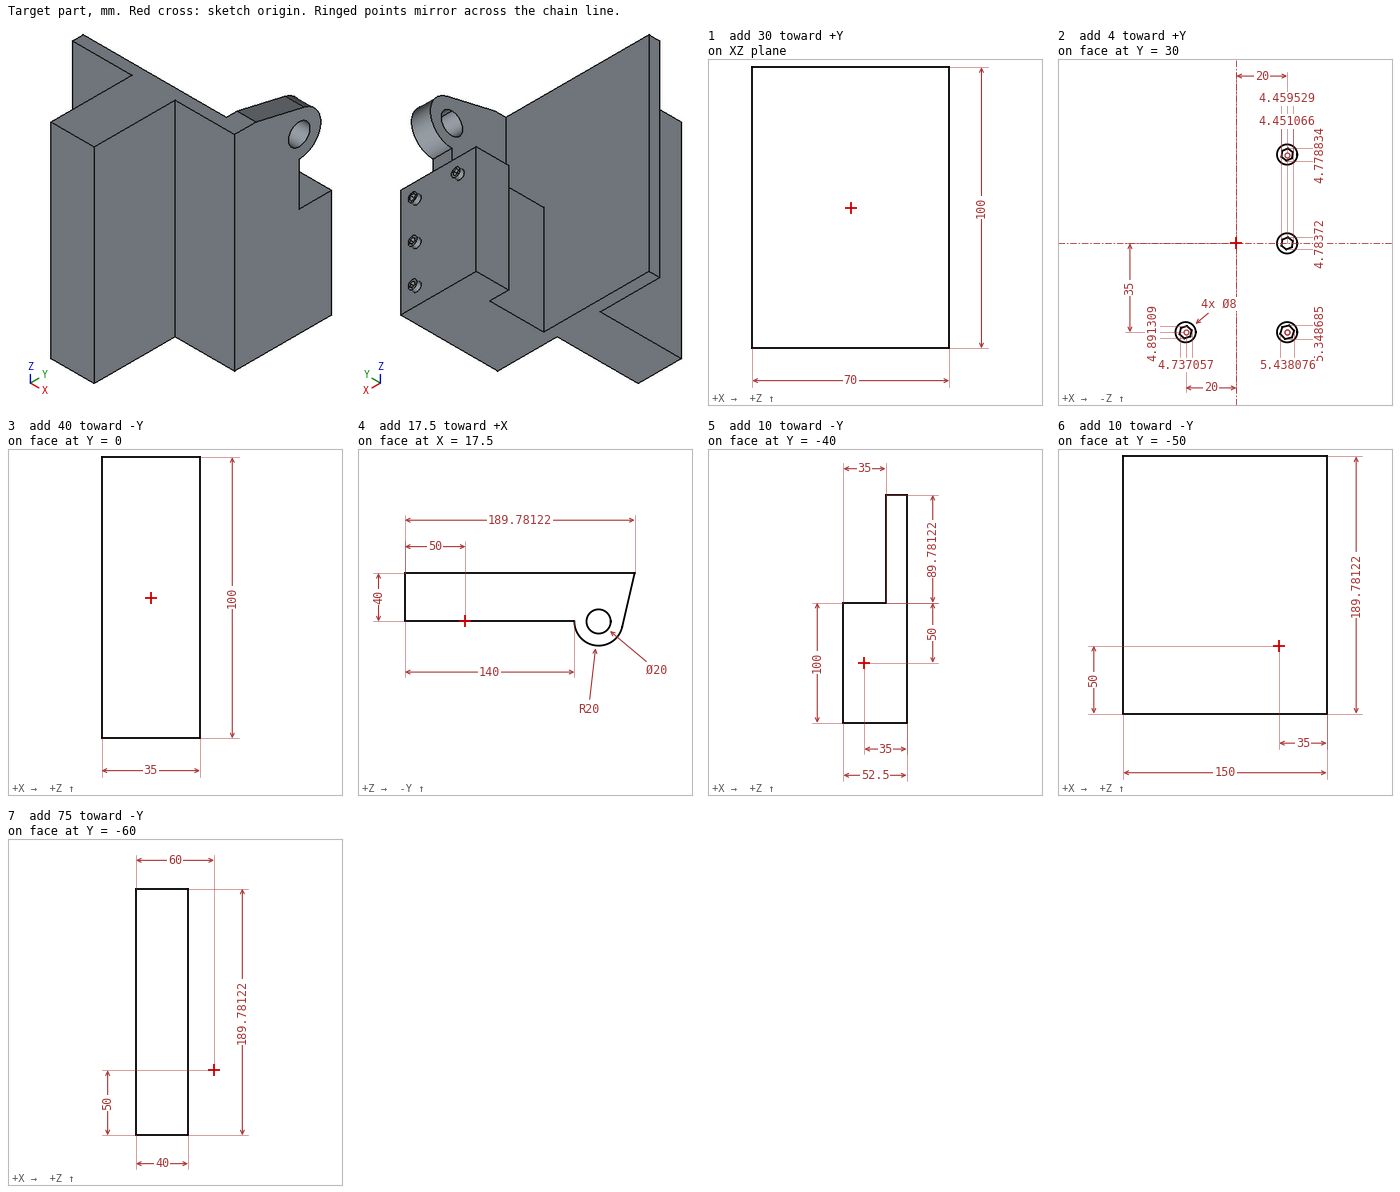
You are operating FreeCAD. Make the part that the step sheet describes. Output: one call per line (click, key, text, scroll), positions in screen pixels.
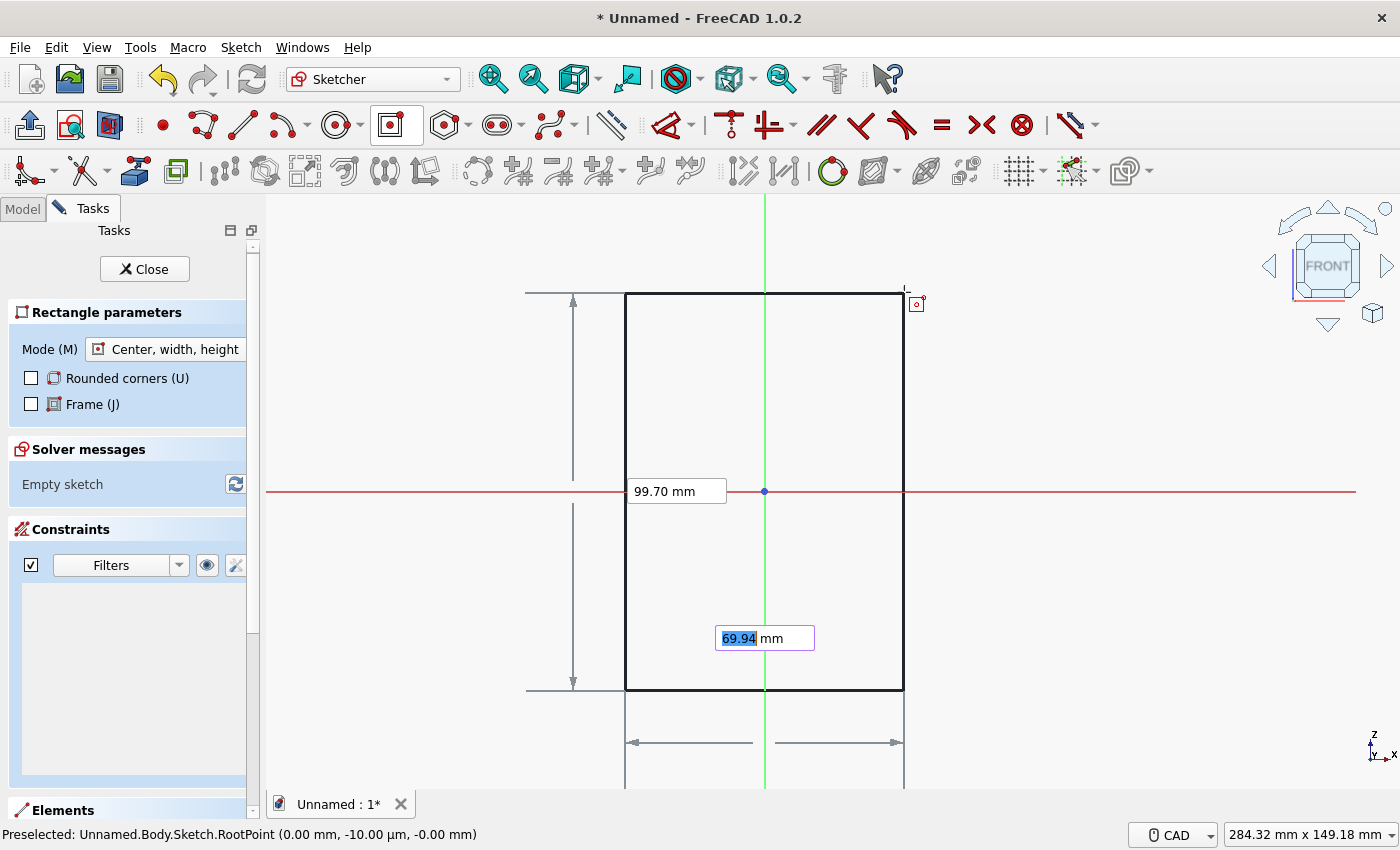
text(70)
key(Tab)
text(100)
key(Return)
key(Escape)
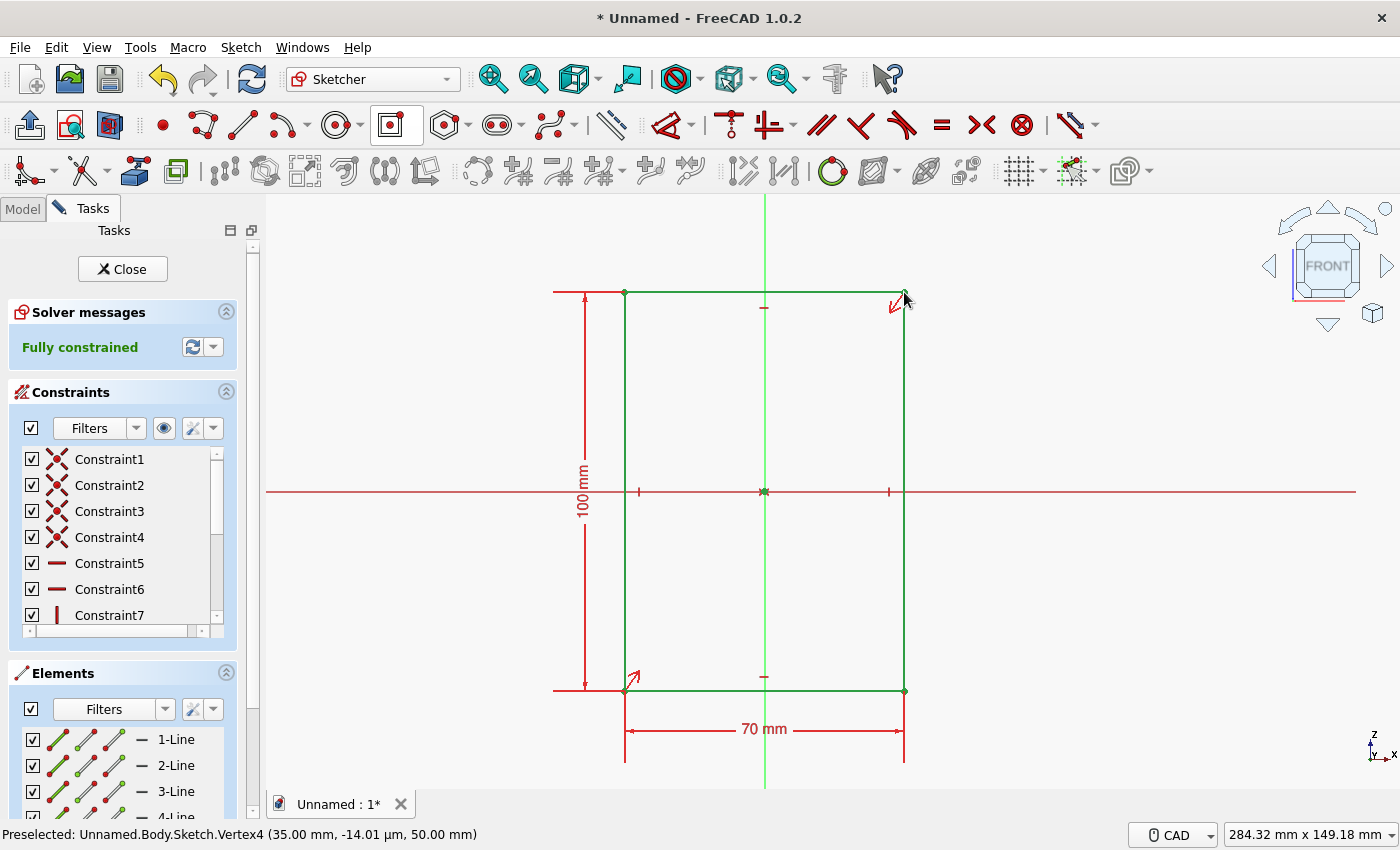
click(123, 269)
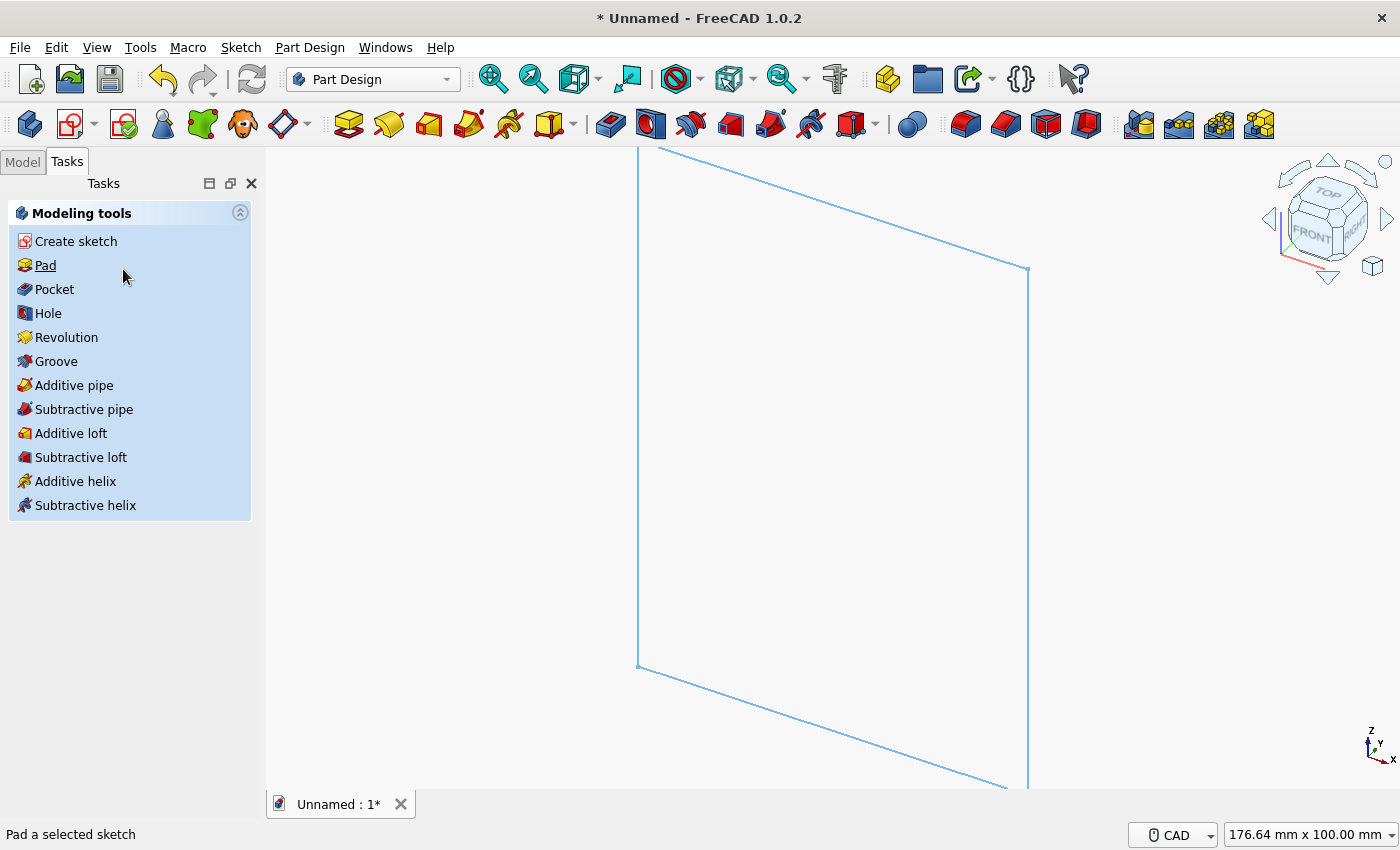
click(350, 124)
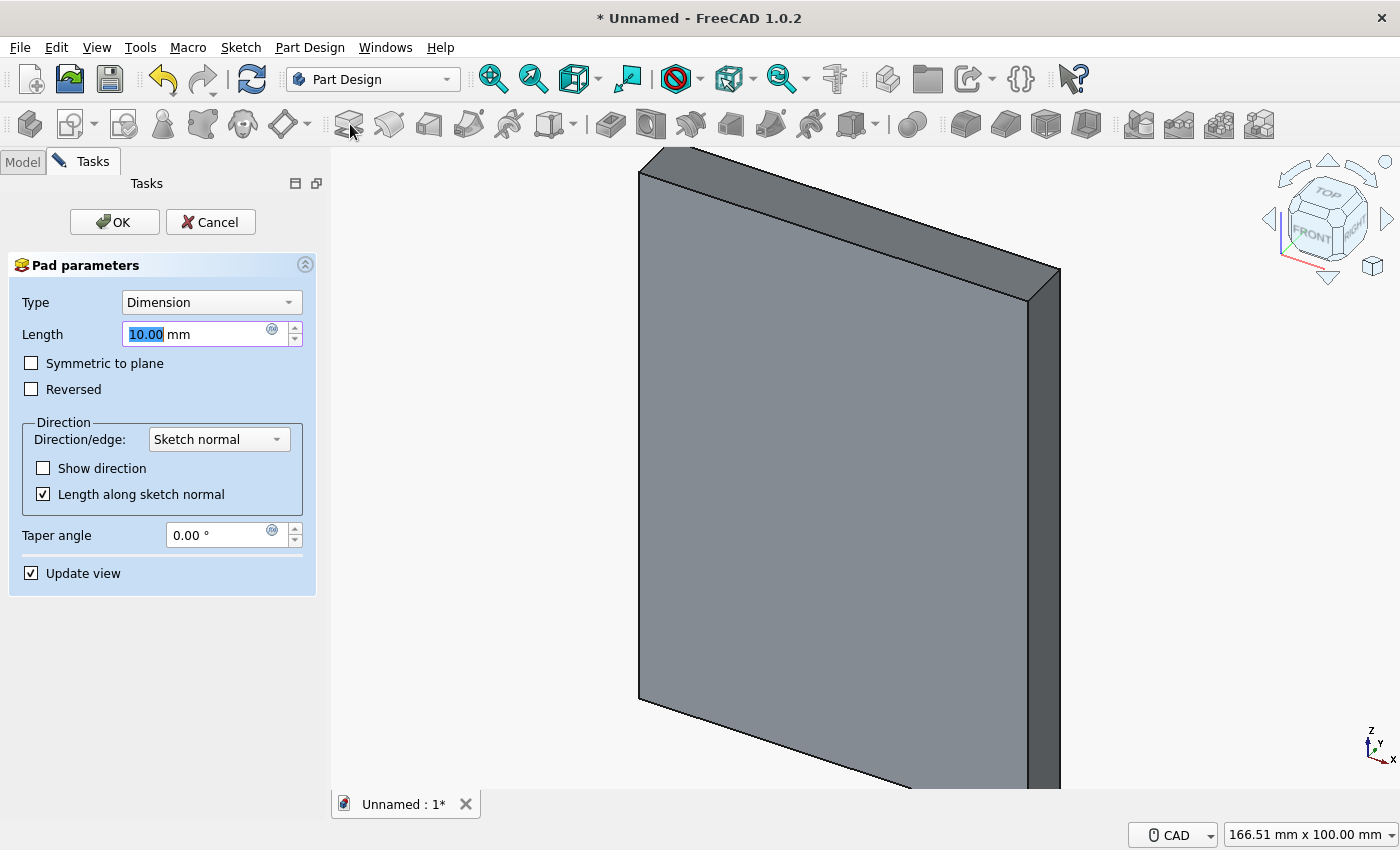
text(30)
key(Tab)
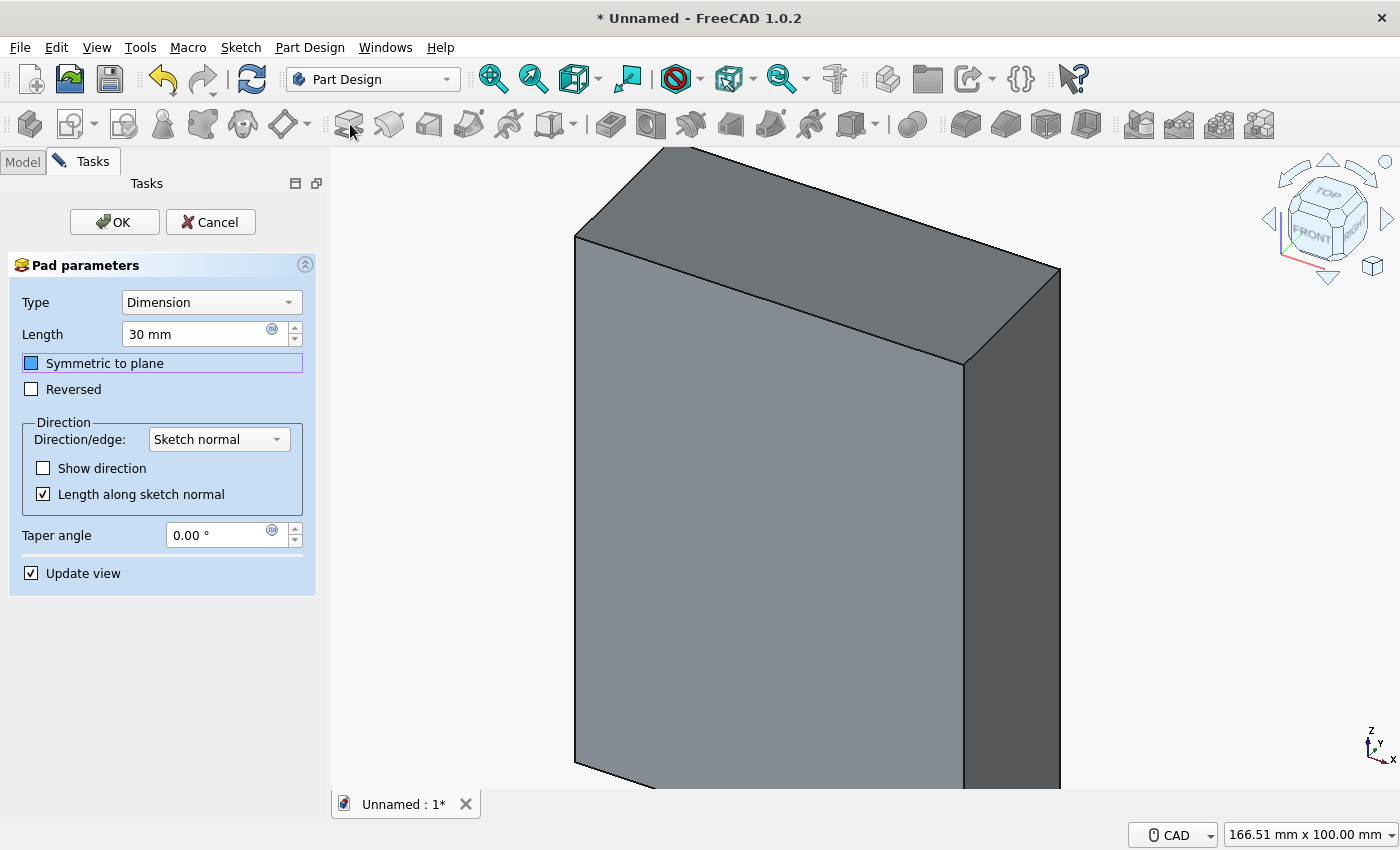
click(30, 389)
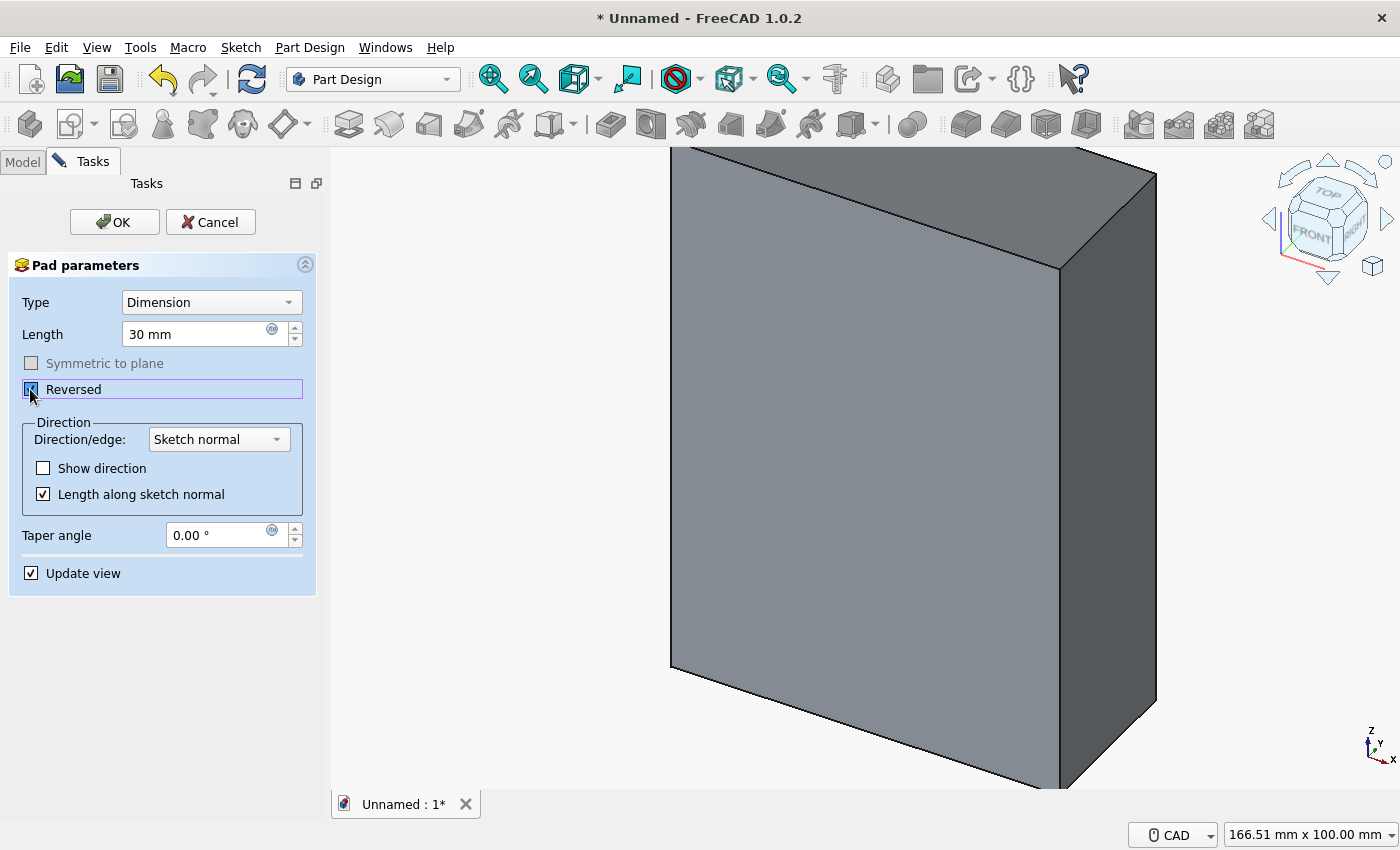
click(115, 222)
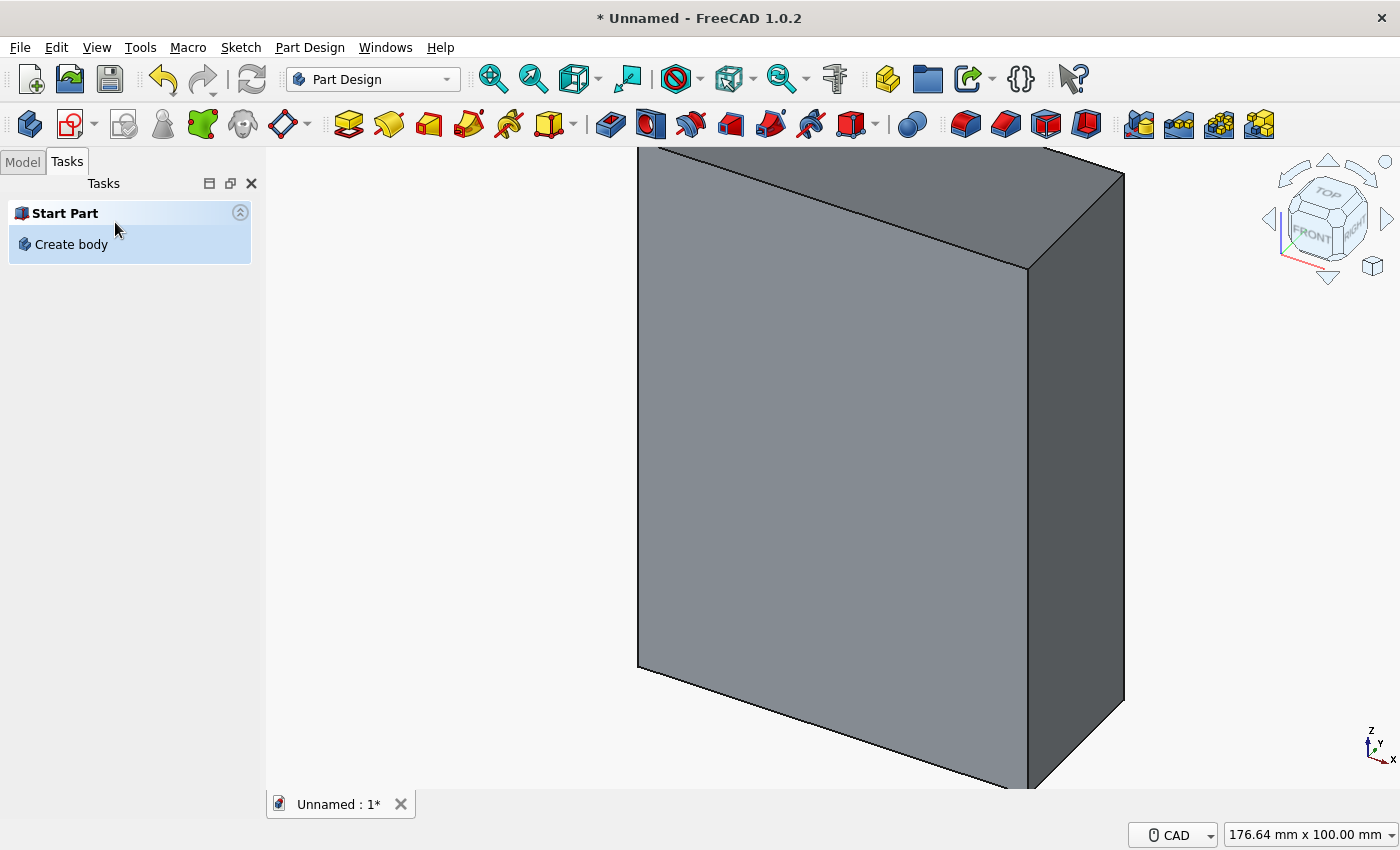
click(494, 80)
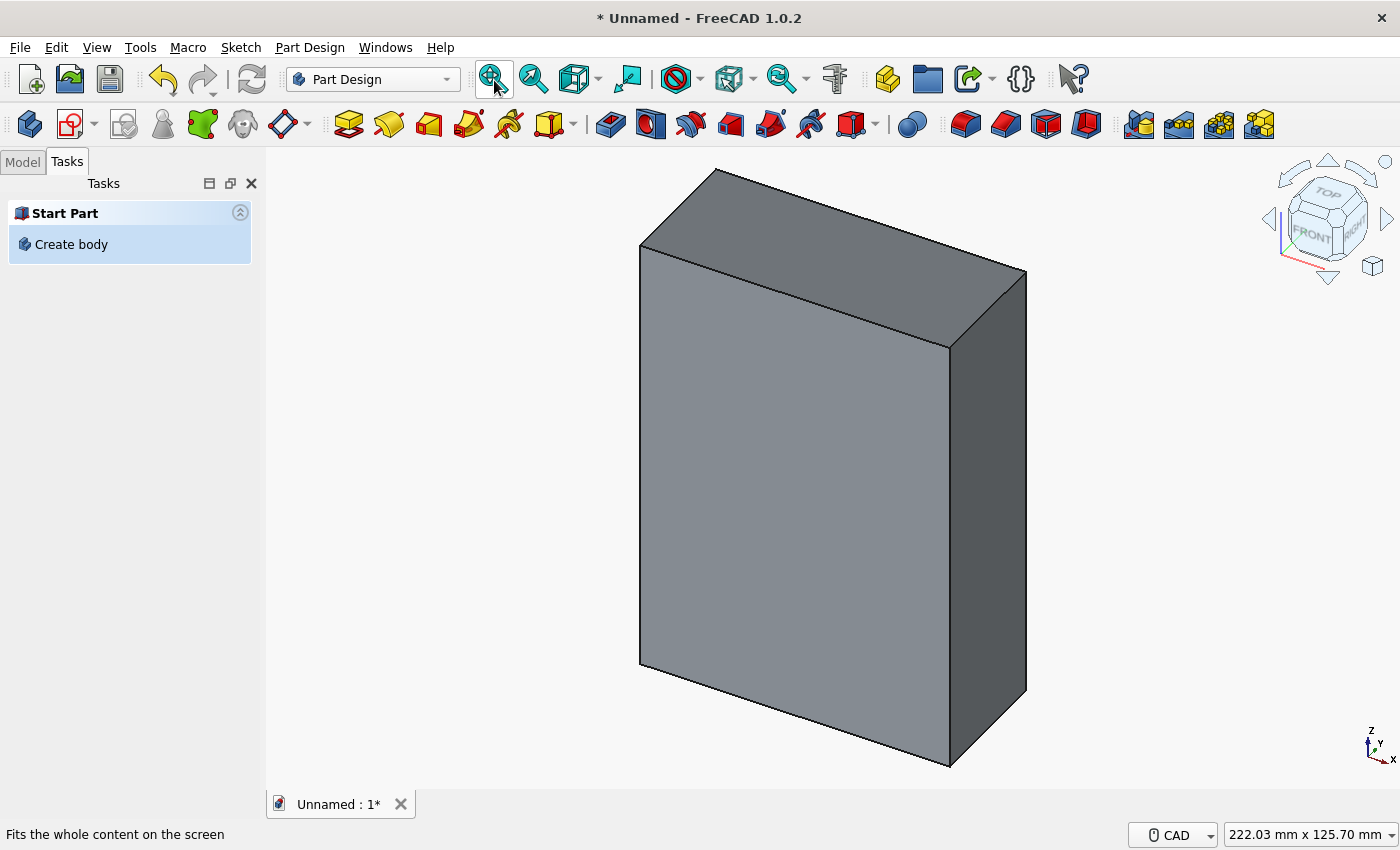
key(4)